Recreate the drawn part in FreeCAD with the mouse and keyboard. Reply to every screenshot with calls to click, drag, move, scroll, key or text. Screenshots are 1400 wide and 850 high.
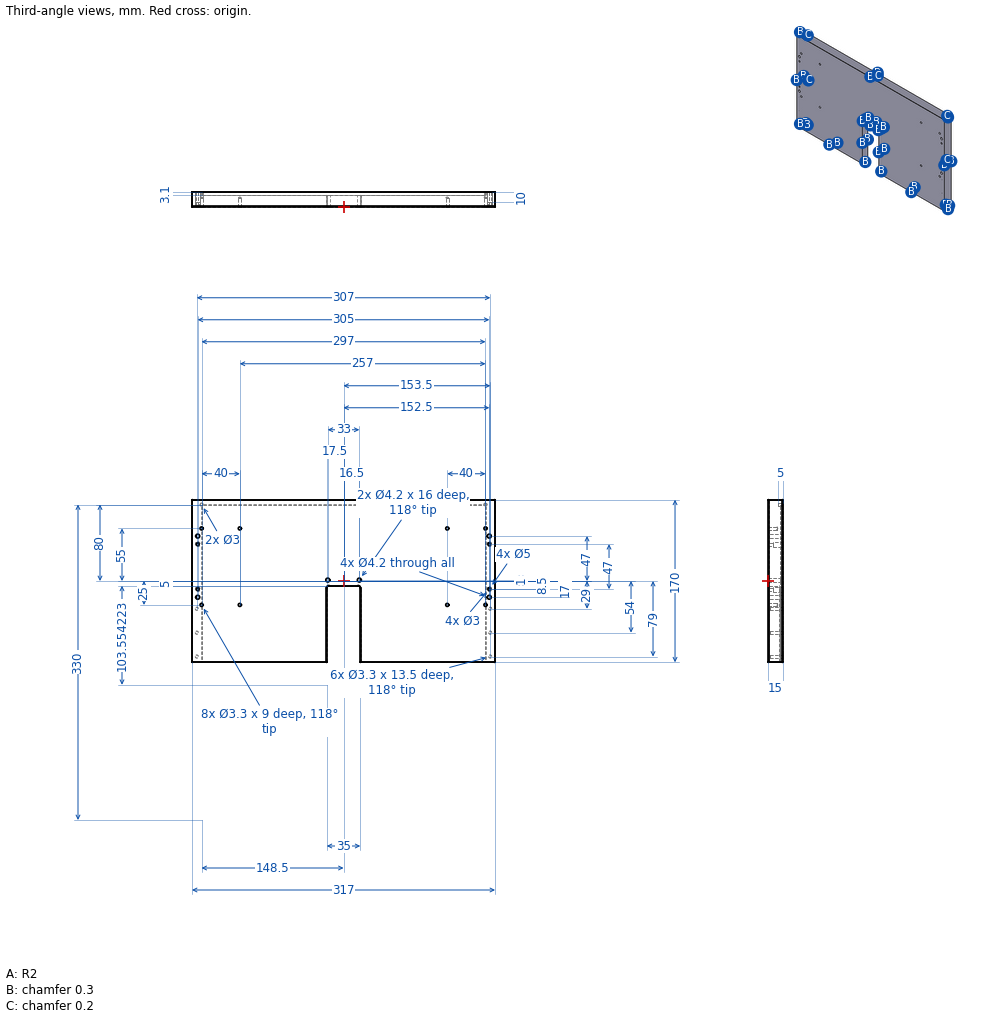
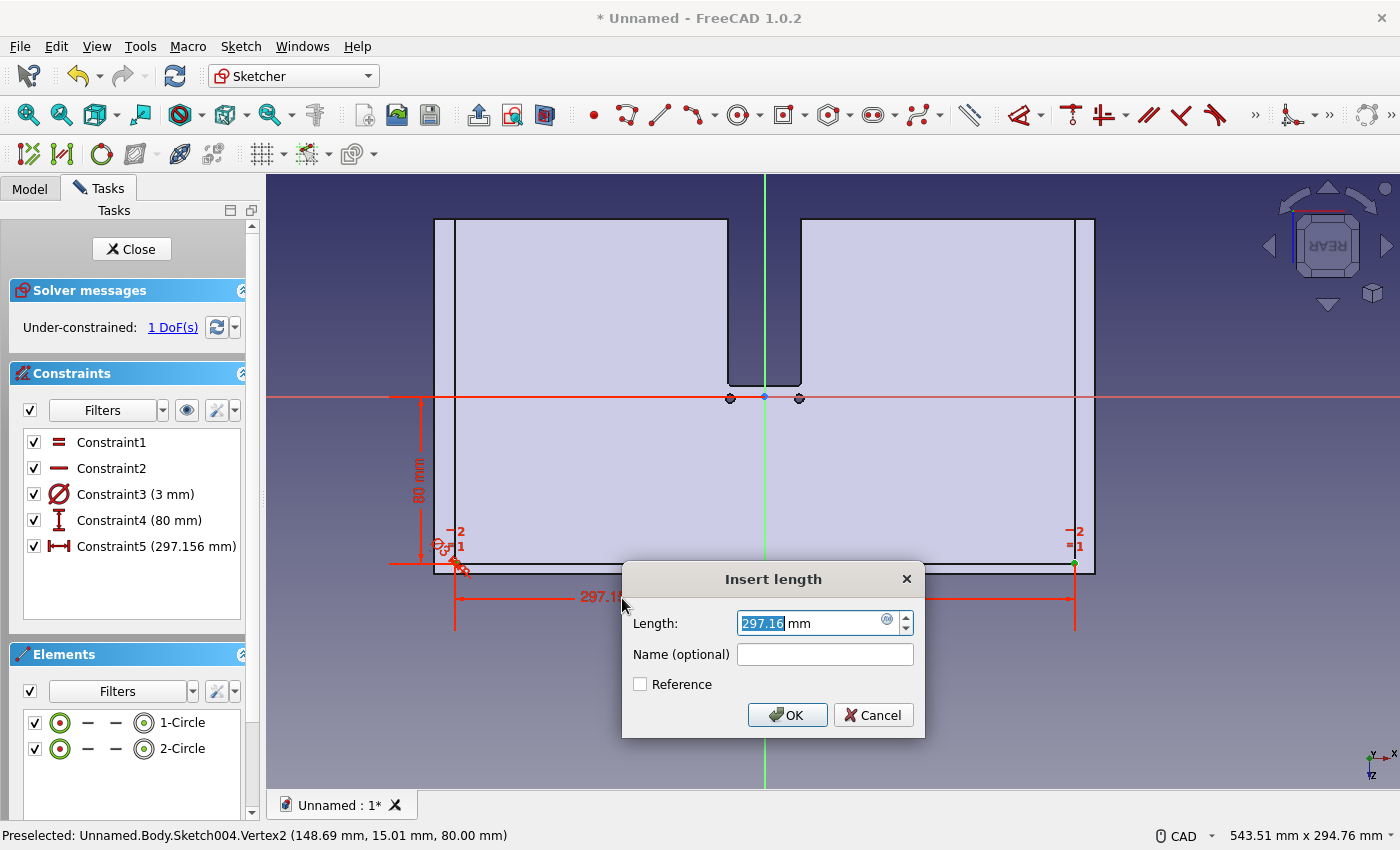
text(297)
key(Return)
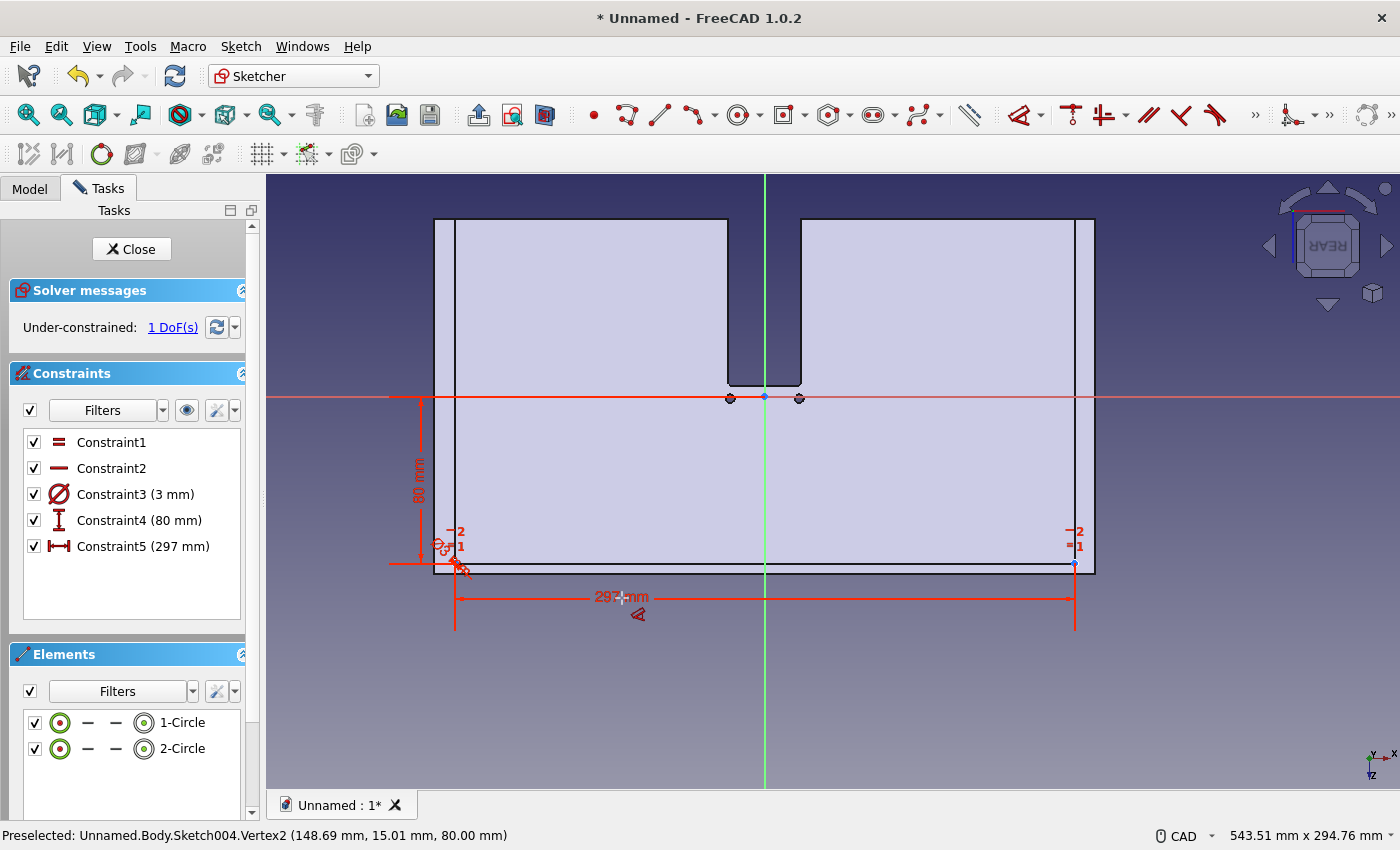
click(455, 564)
click(610, 363)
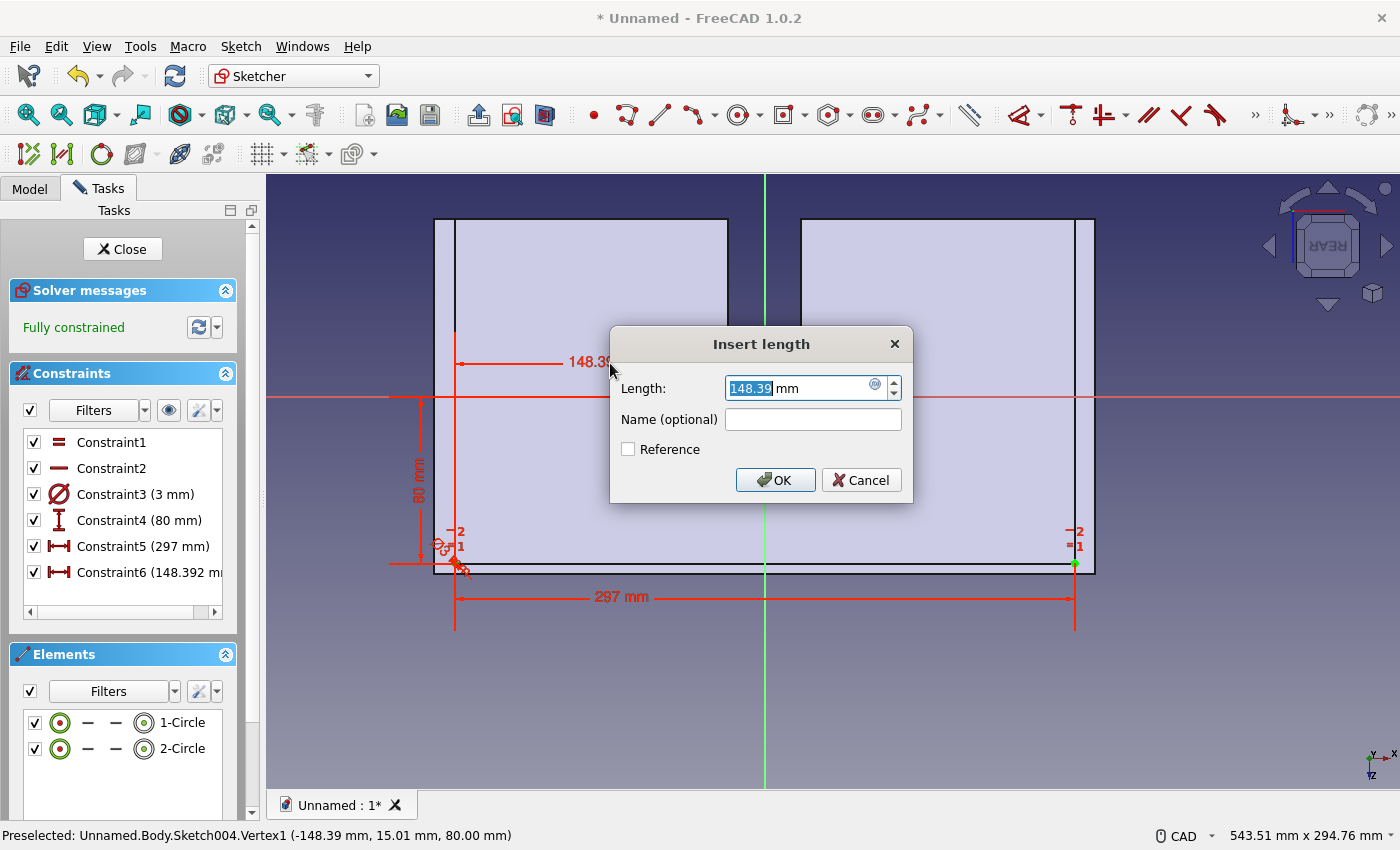
text(148.5)
key(Return)
key(Escape)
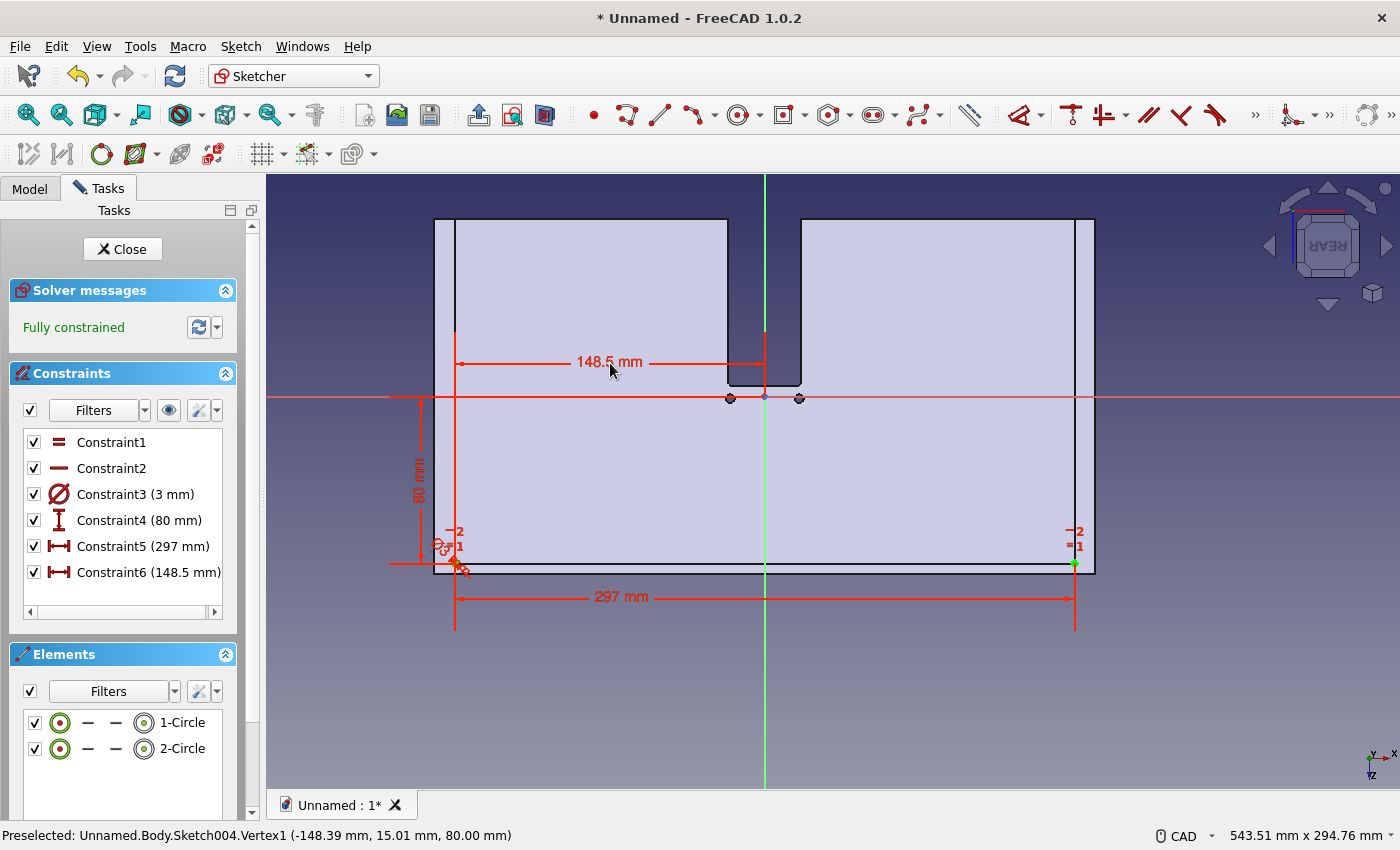
click(123, 249)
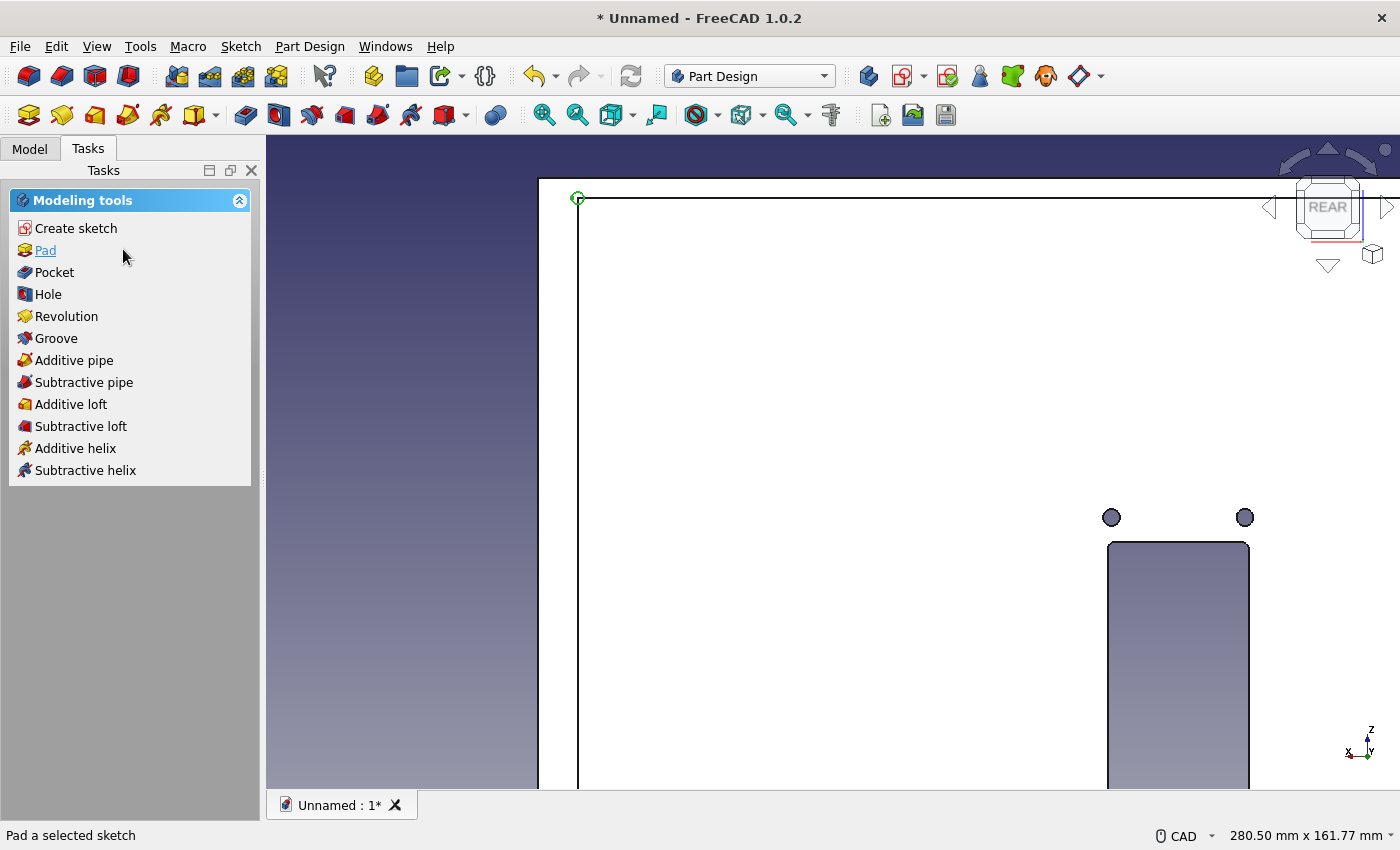
click(246, 116)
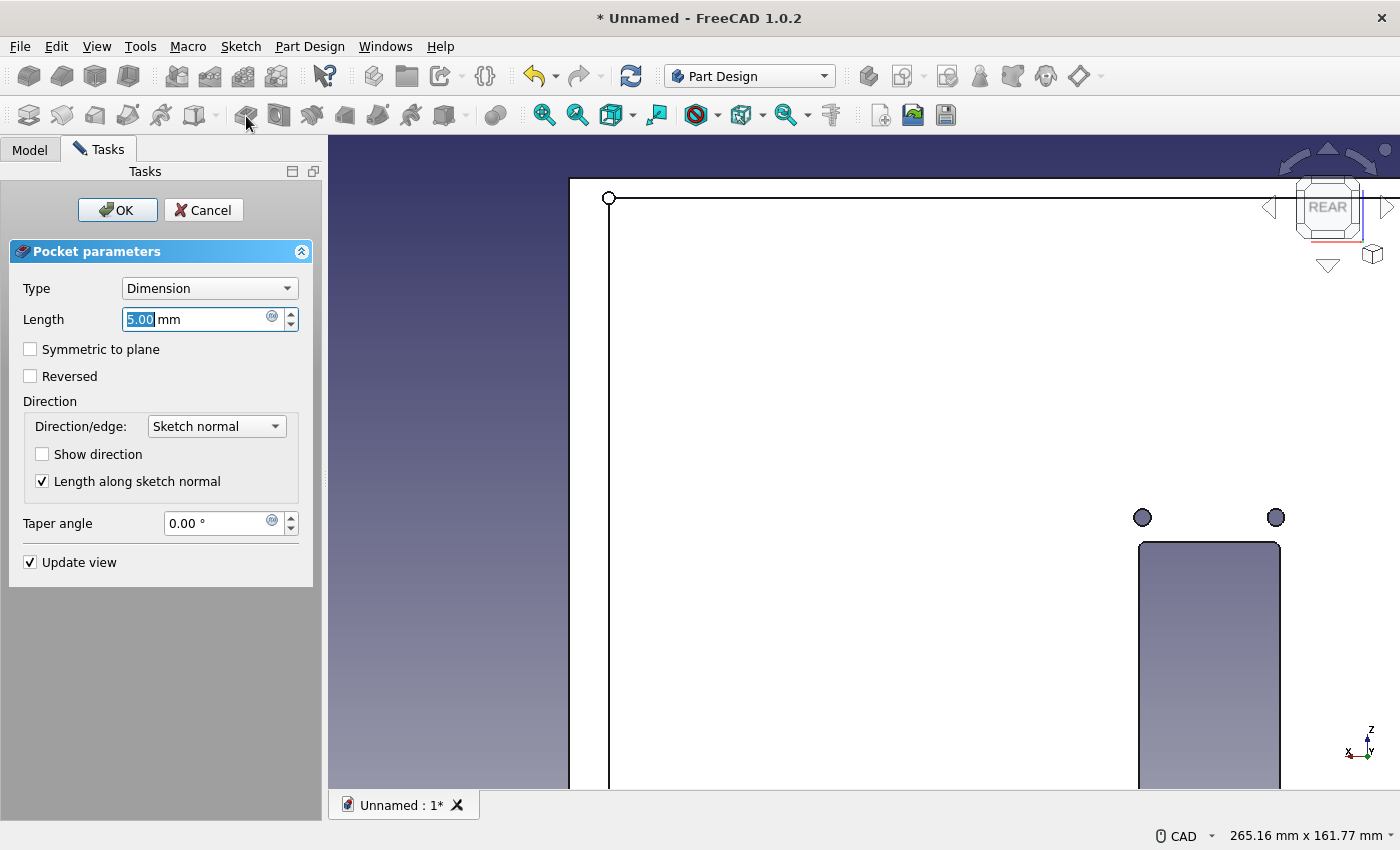
text(5)
key(Tab)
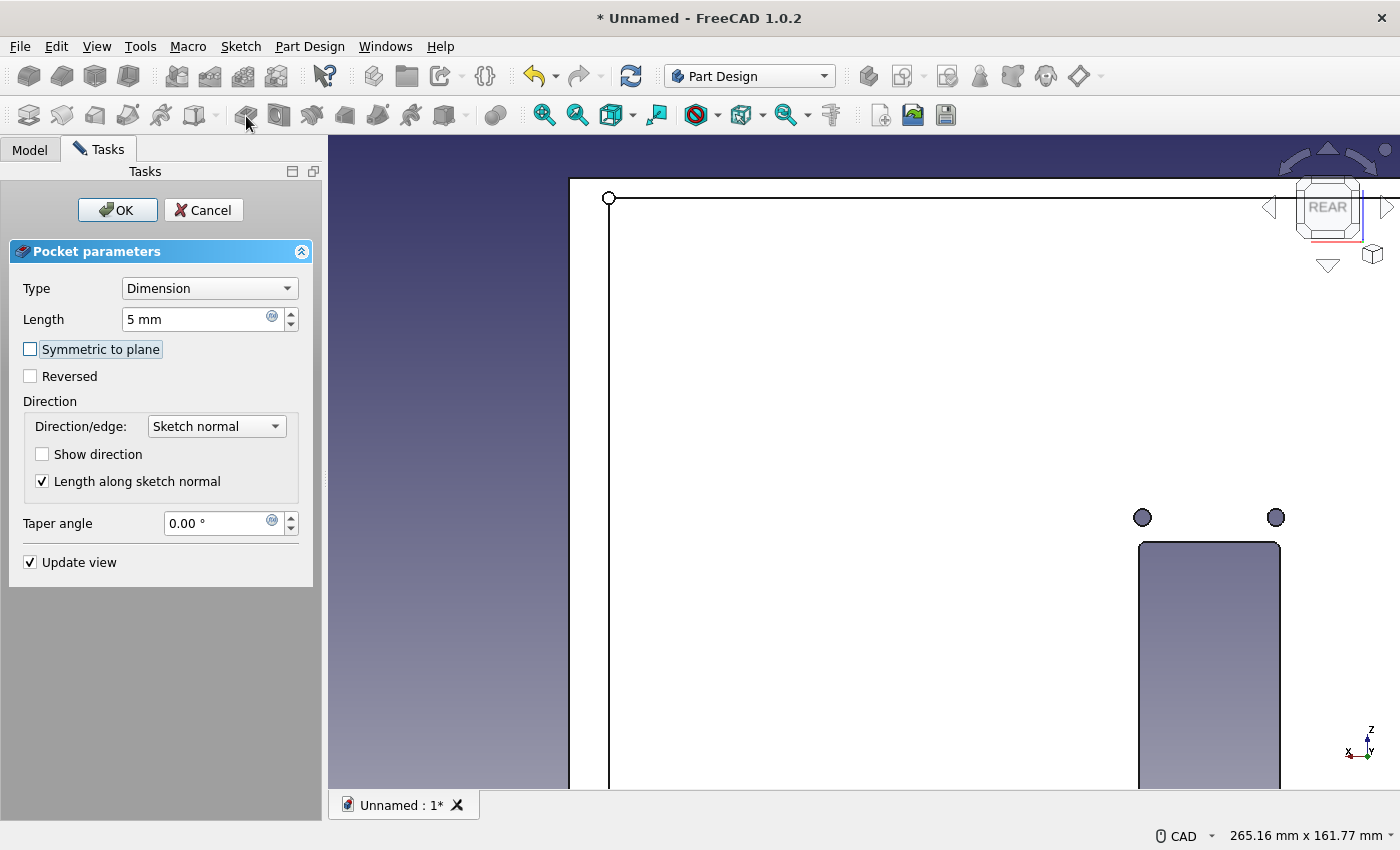
click(118, 210)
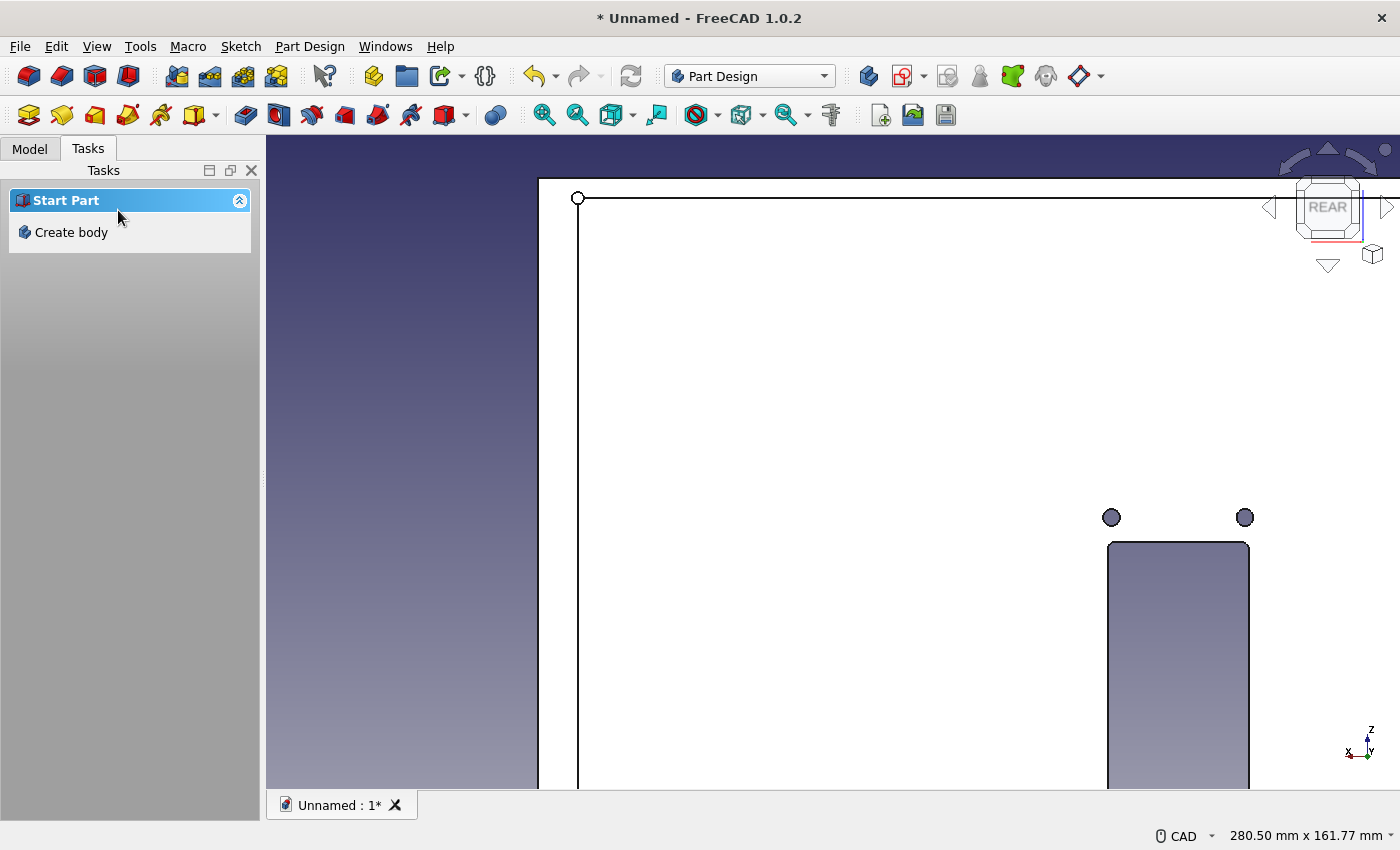
key(v)
key(f)